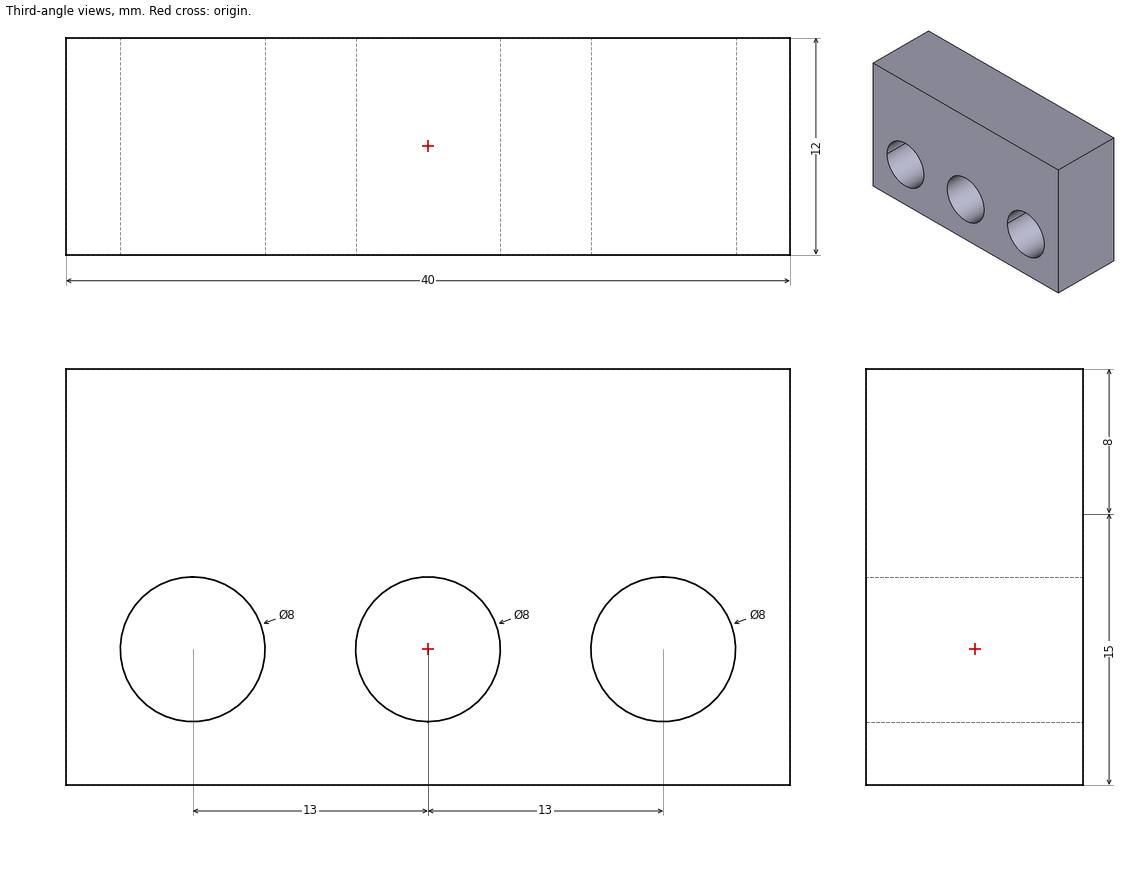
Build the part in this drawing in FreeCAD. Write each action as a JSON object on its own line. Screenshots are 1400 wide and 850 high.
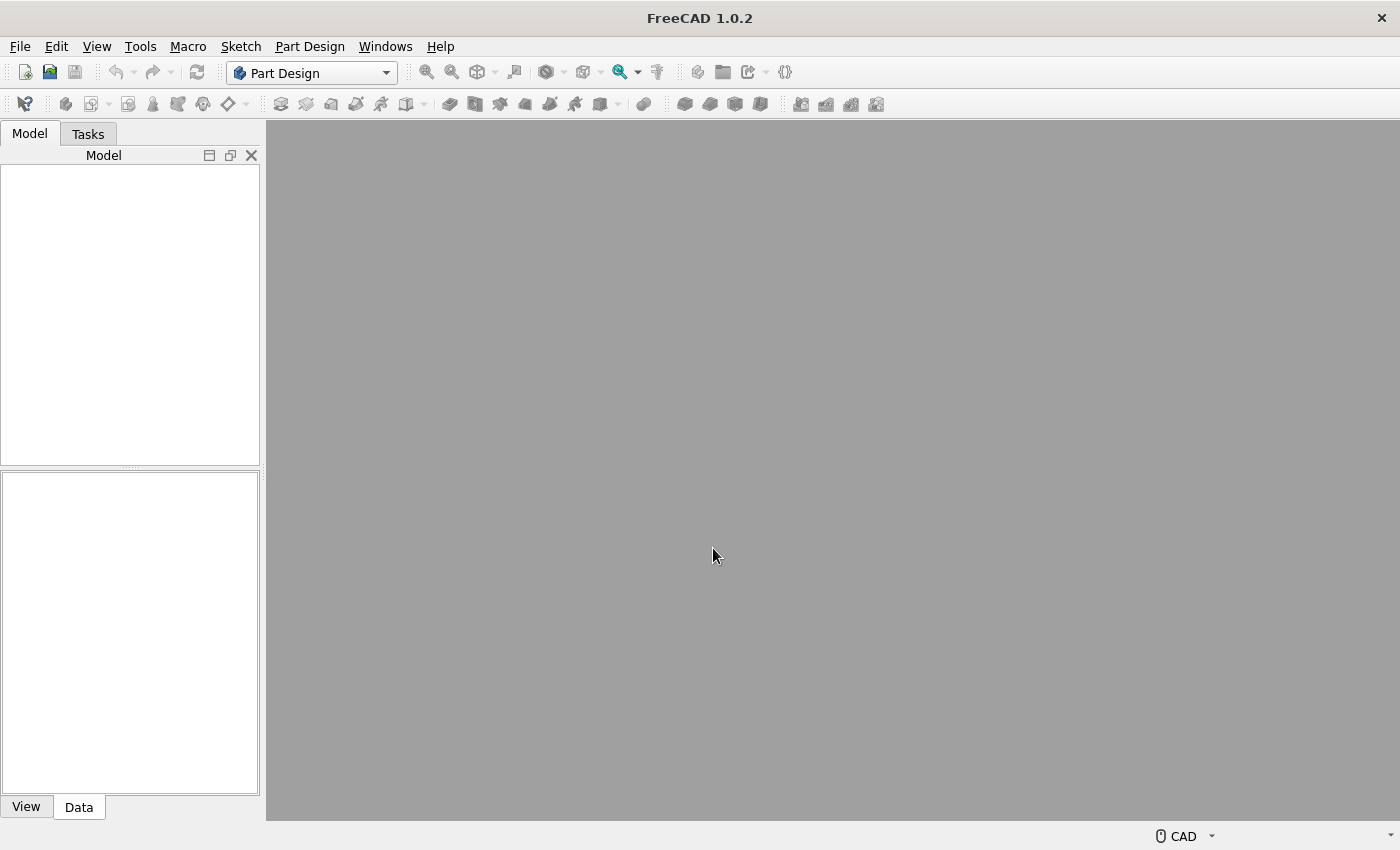
{"action": "key", "text": "ctrl+n"}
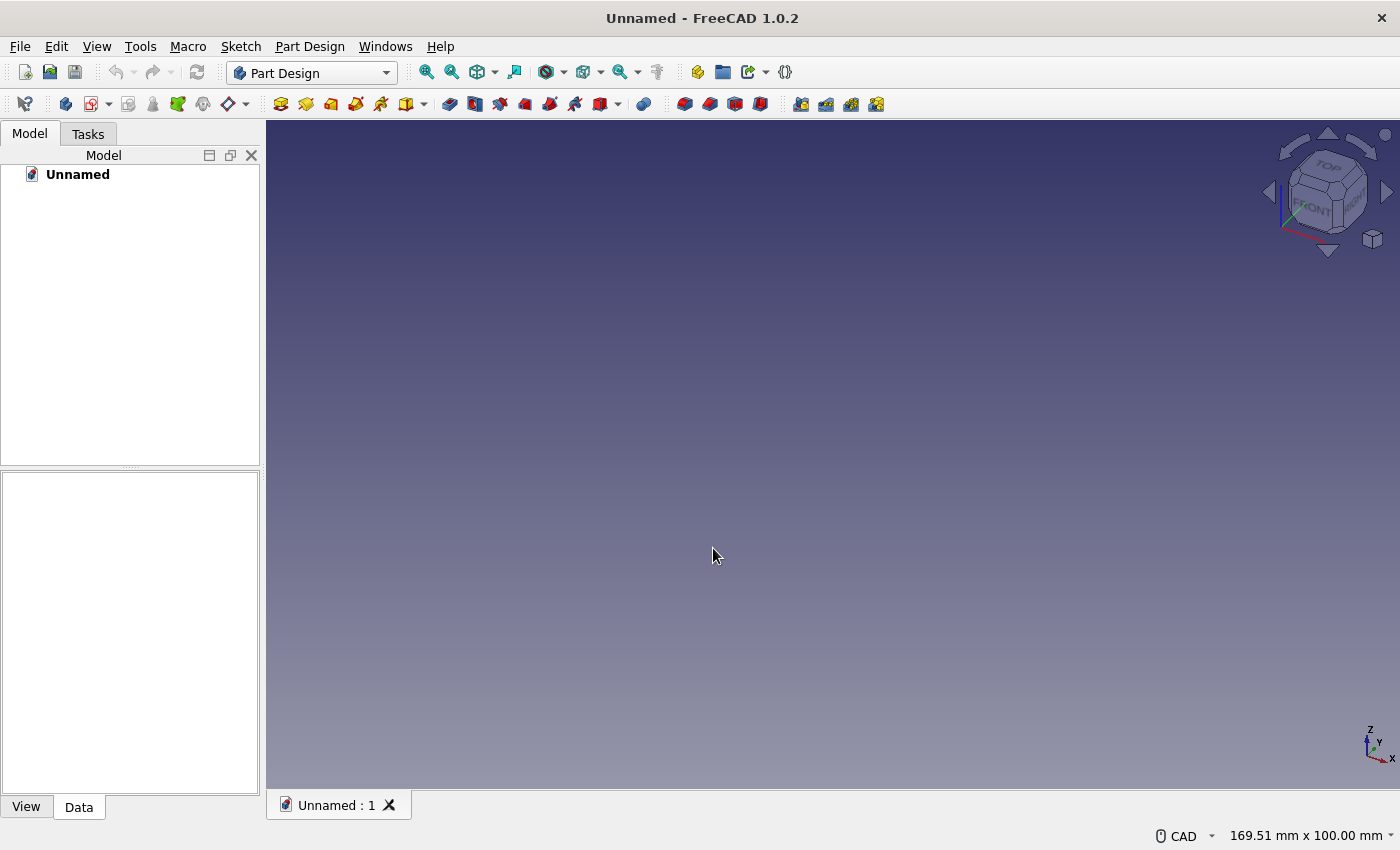
{"action": "left_click", "coordinate": [90, 104]}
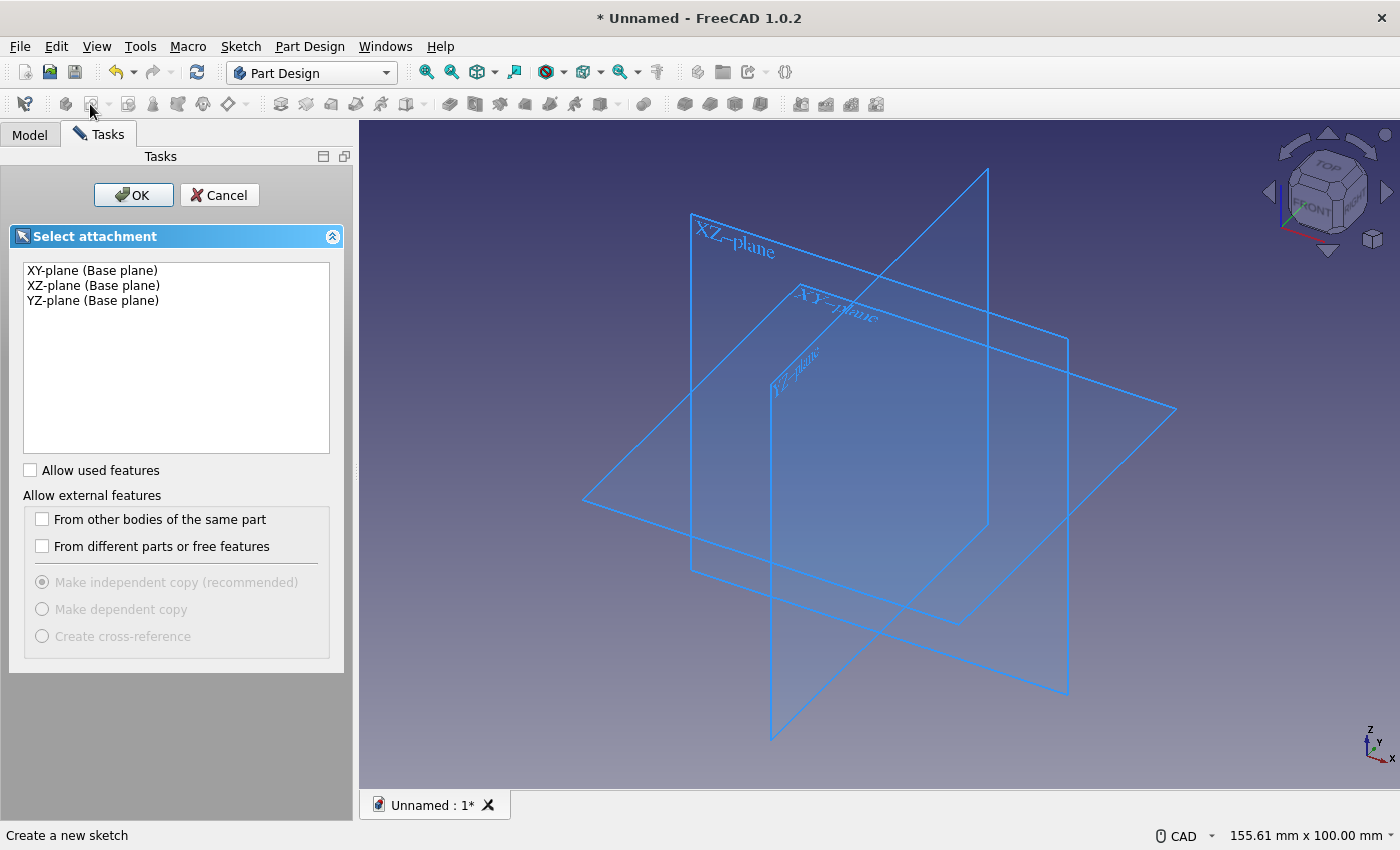
{"action": "left_click", "coordinate": [84, 270]}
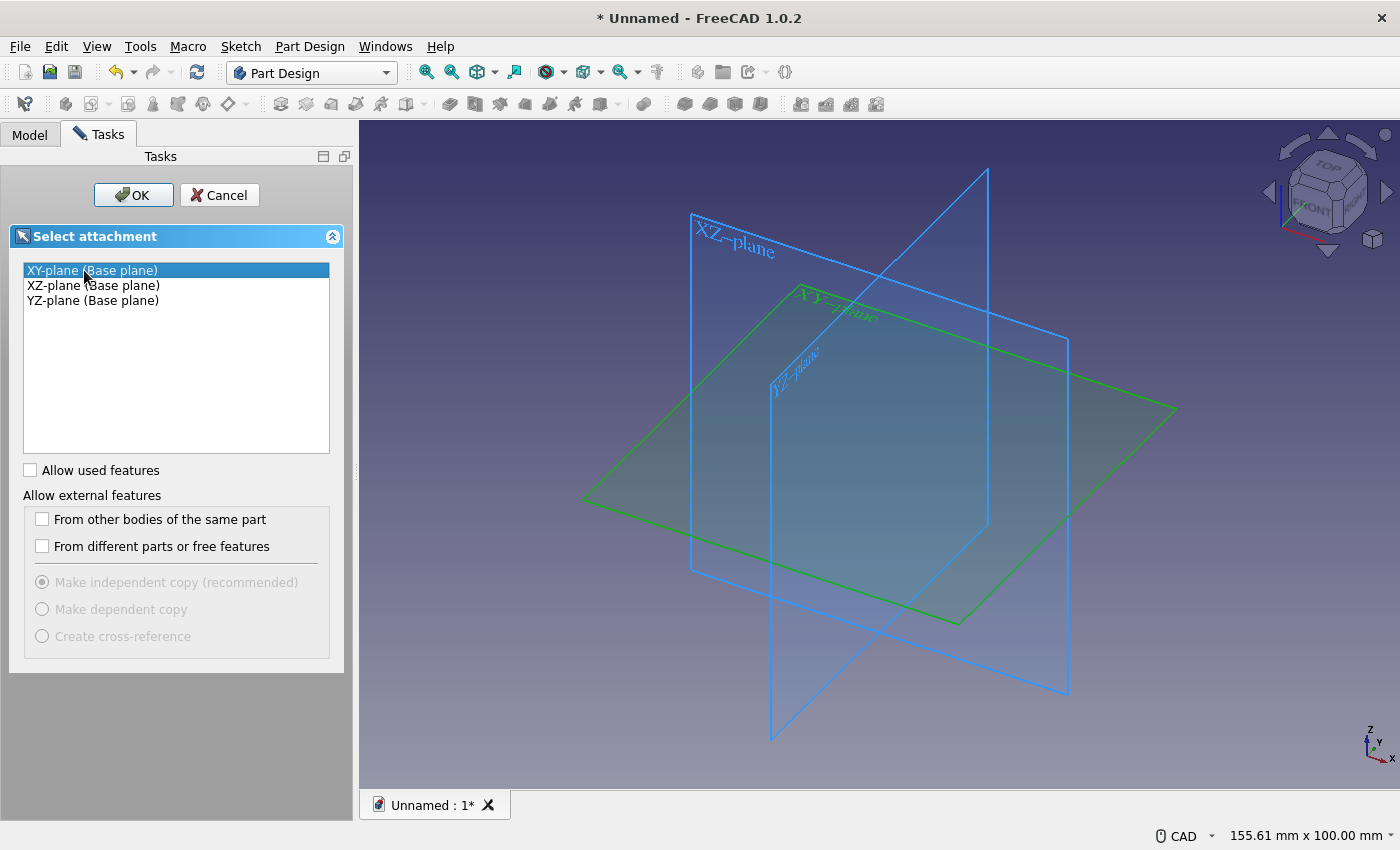
{"action": "left_click", "coordinate": [134, 195]}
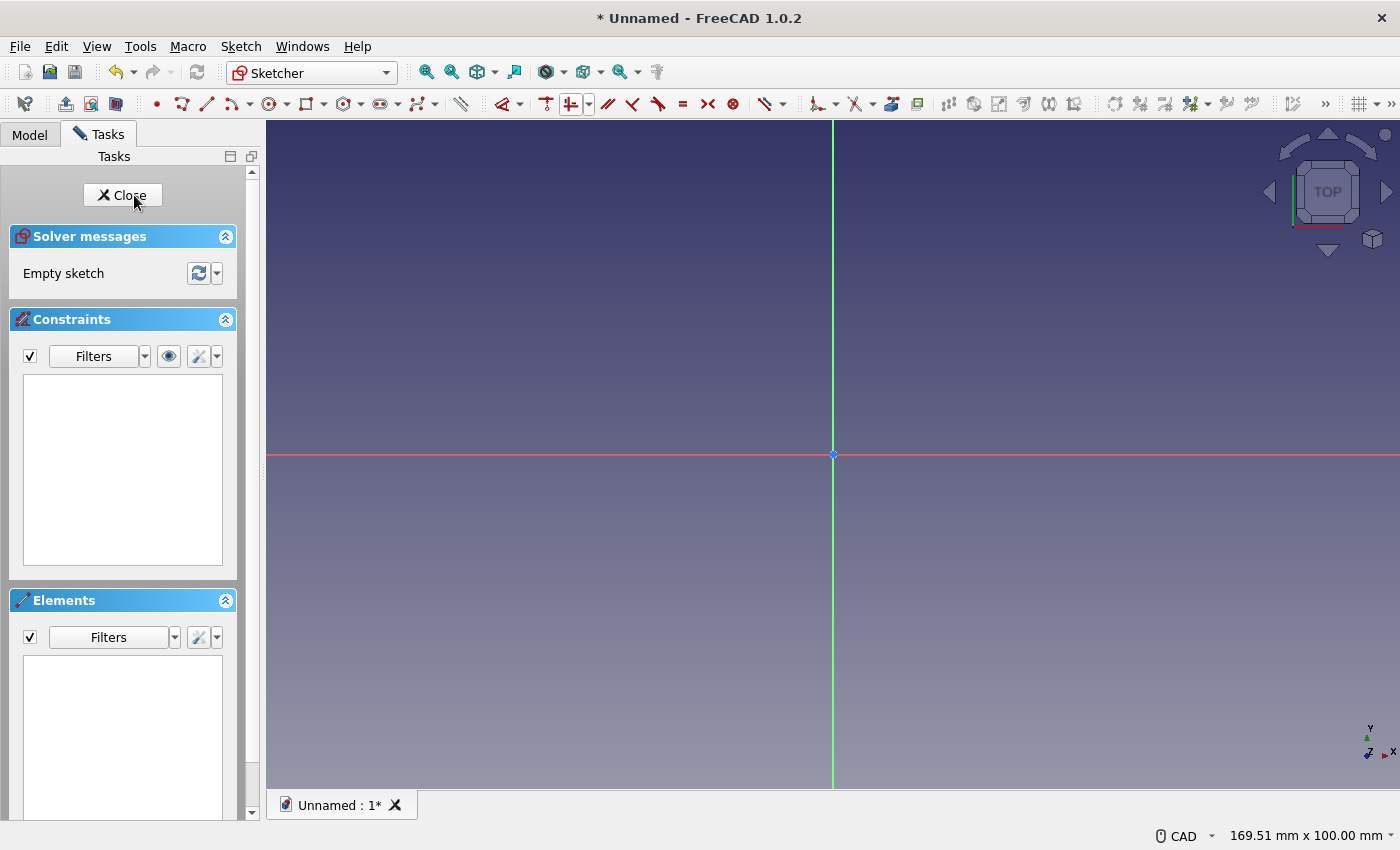
{"action": "scroll", "coordinate": [873, 454], "scroll_direction": "up", "scroll_amount": 5}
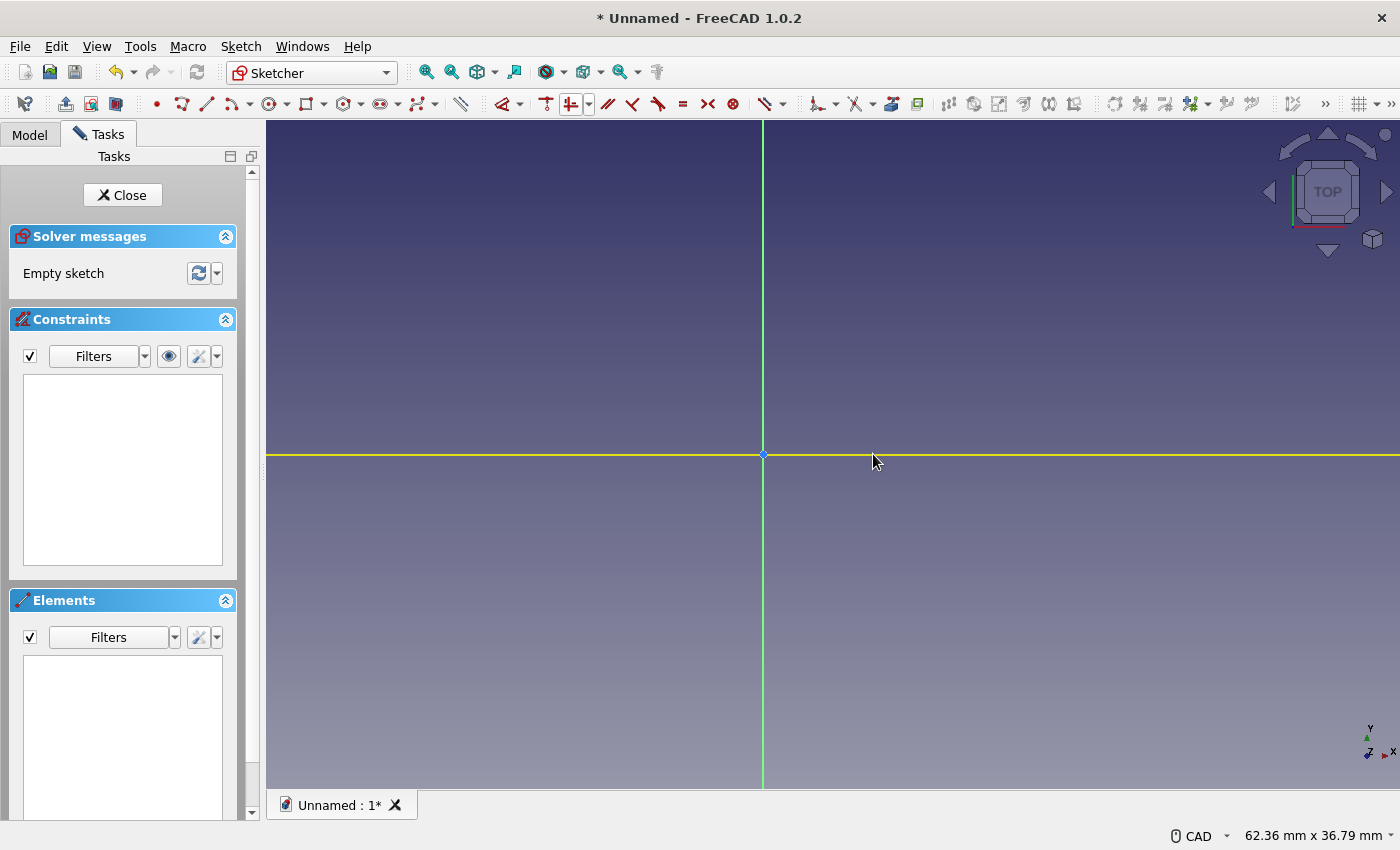
{"action": "key", "text": "g v"}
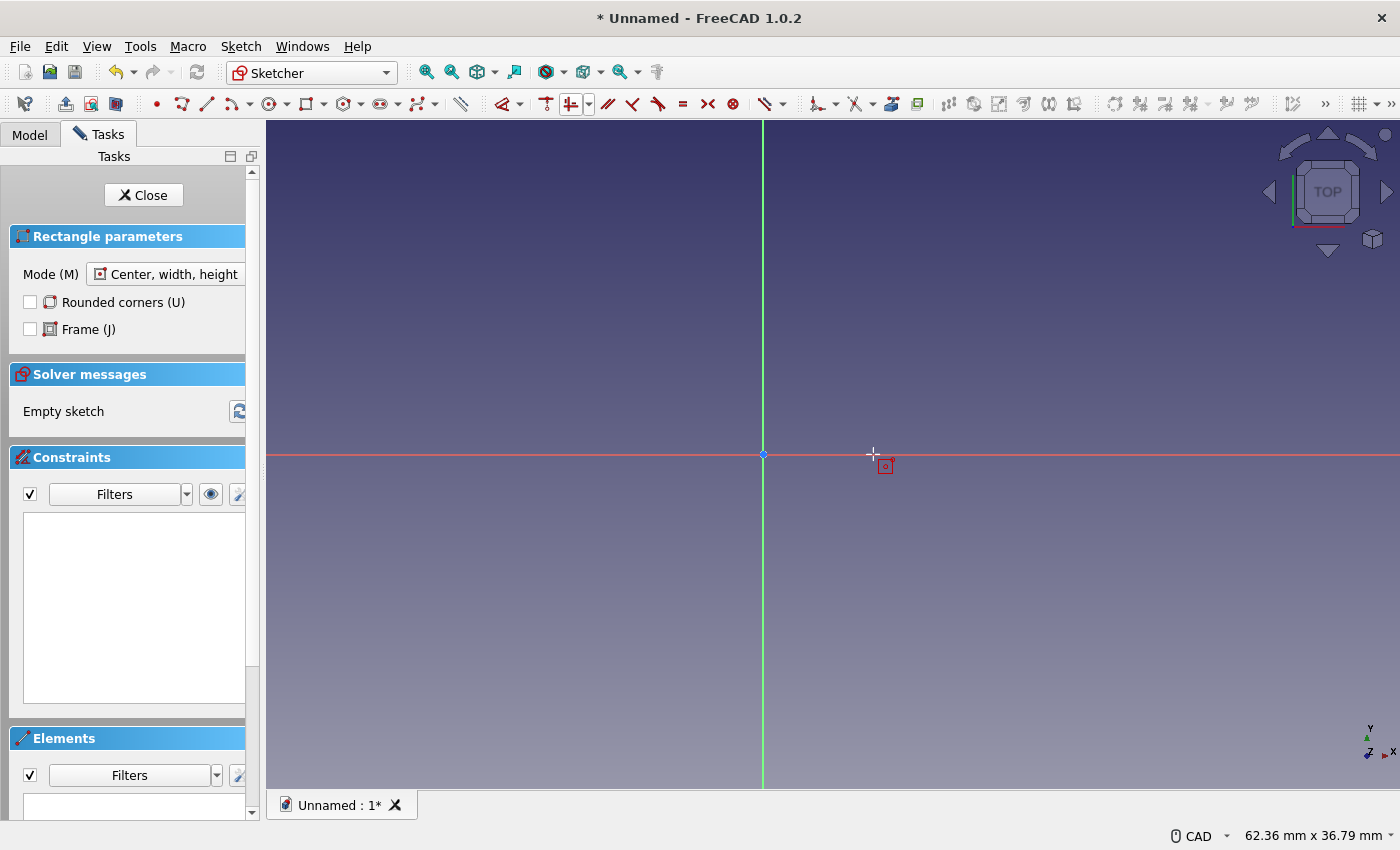
{"action": "left_click", "coordinate": [763, 454]}
{"action": "left_click", "coordinate": [1127, 345]}
{"action": "key", "text": "Escape"}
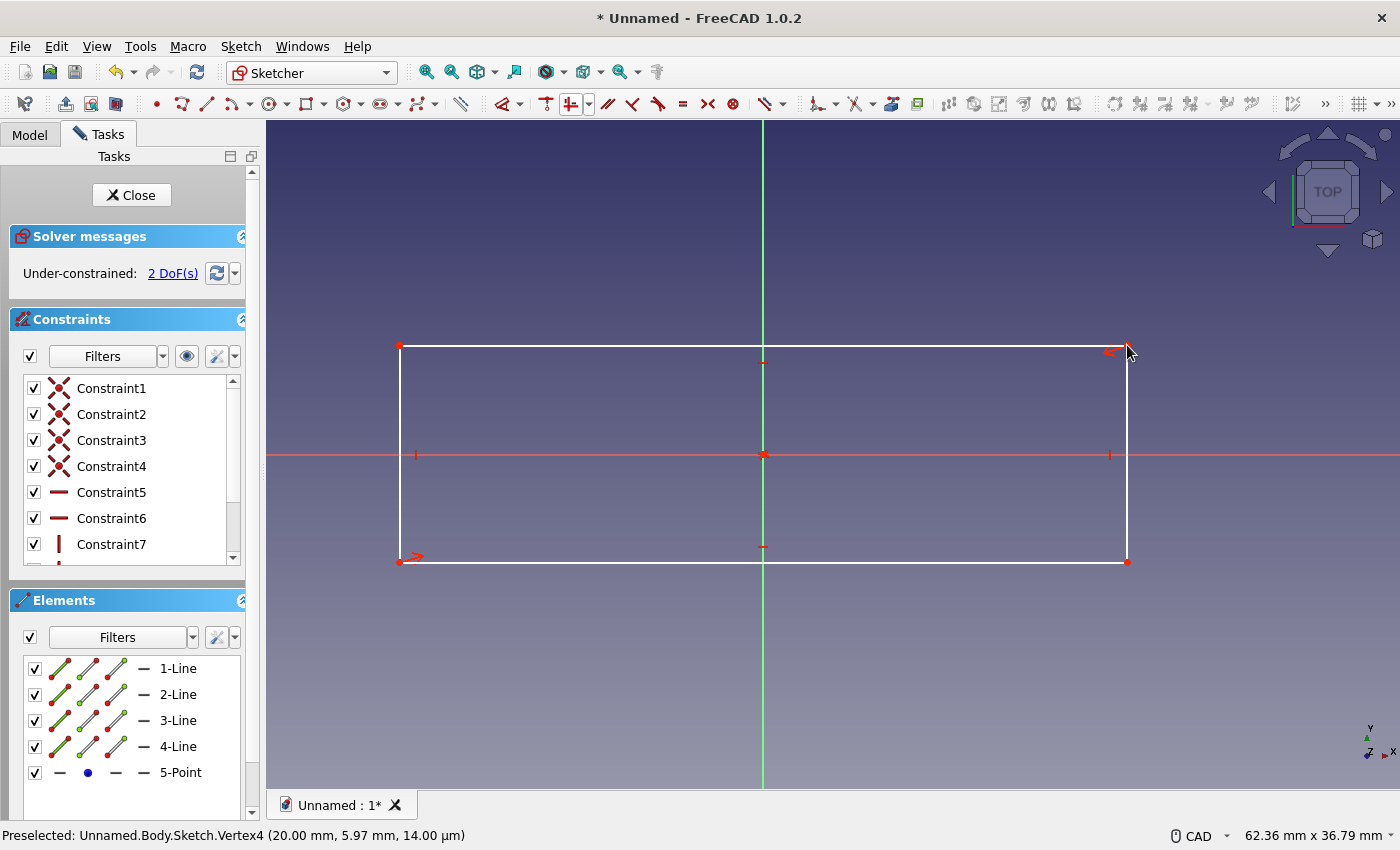
{"action": "left_click", "coordinate": [502, 104]}